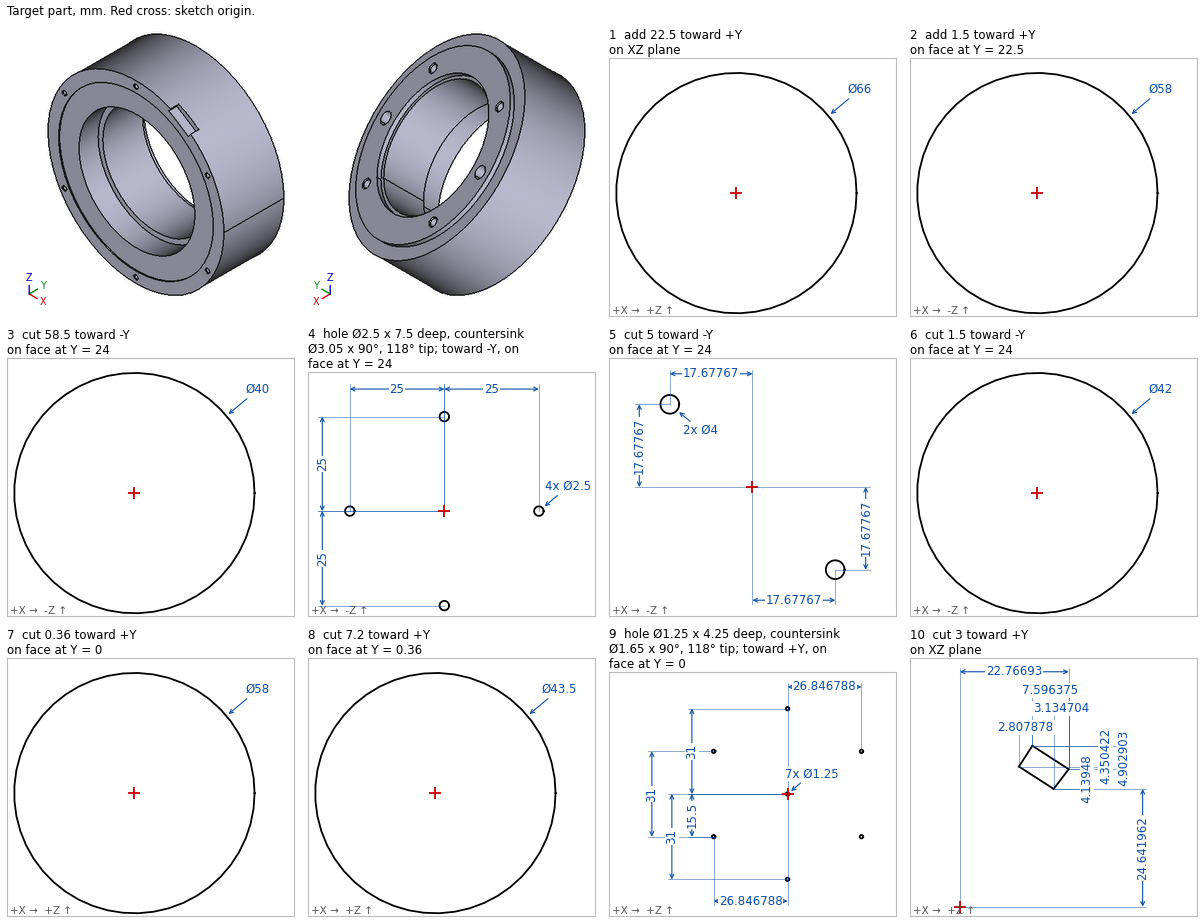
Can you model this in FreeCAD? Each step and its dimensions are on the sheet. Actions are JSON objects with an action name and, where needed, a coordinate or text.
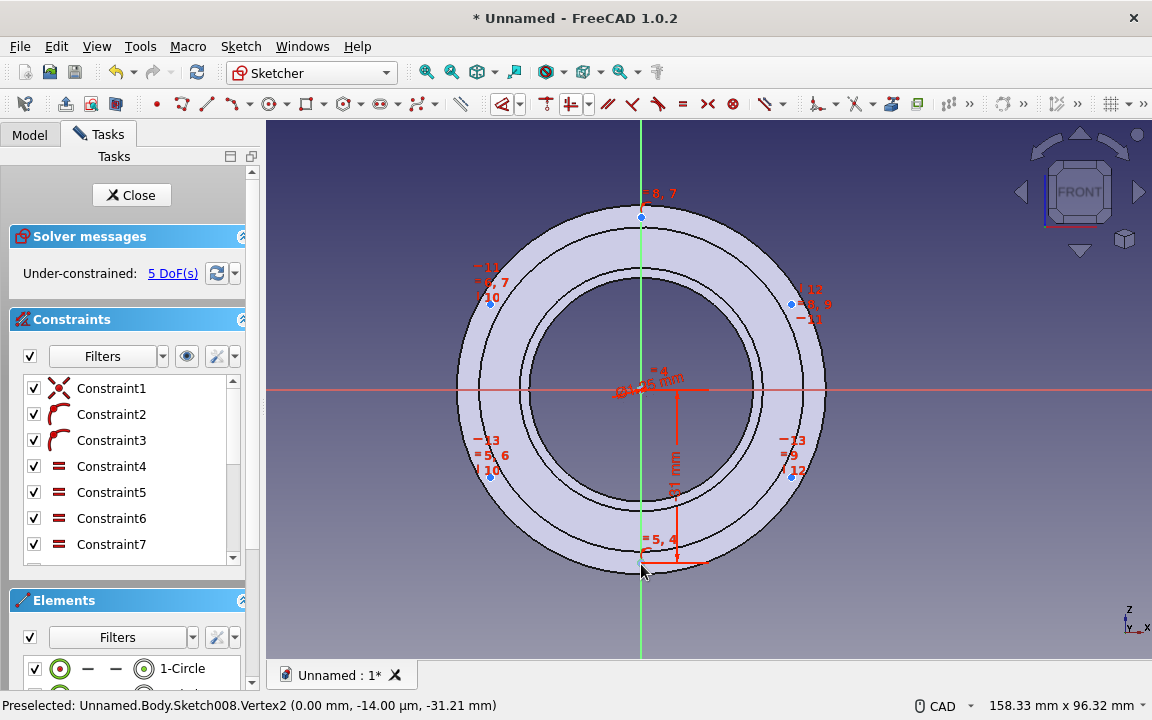
{"action": "left_click", "coordinate": [641, 217]}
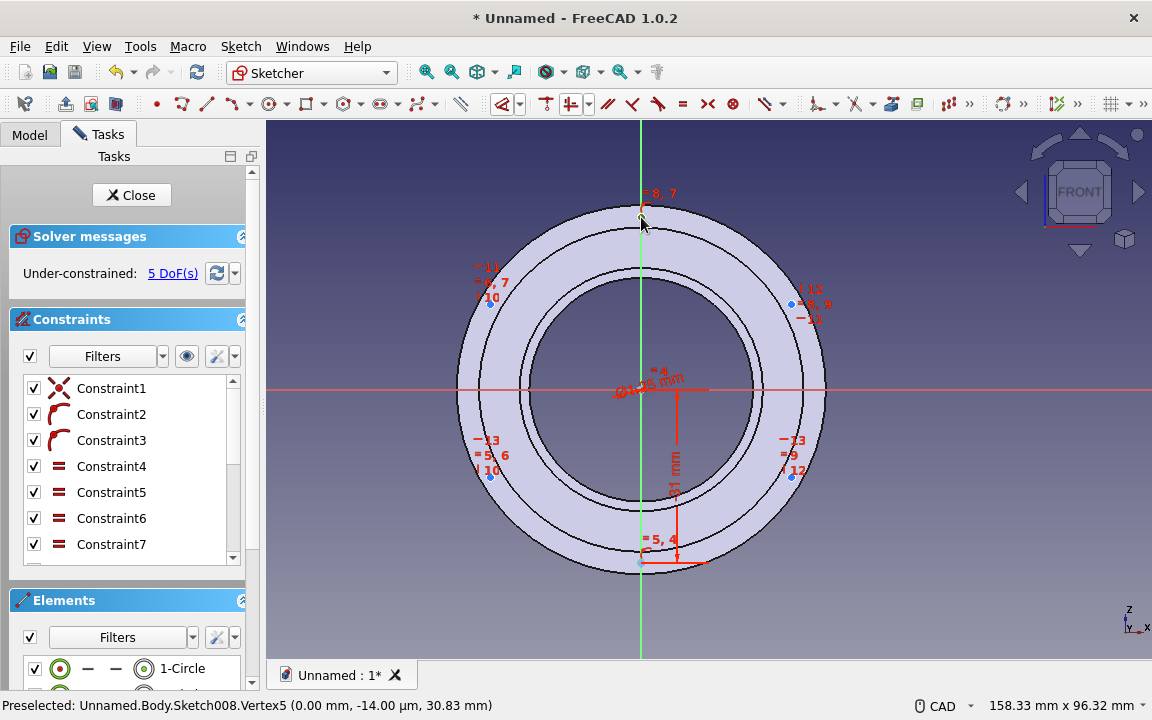
{"action": "key", "text": "i"}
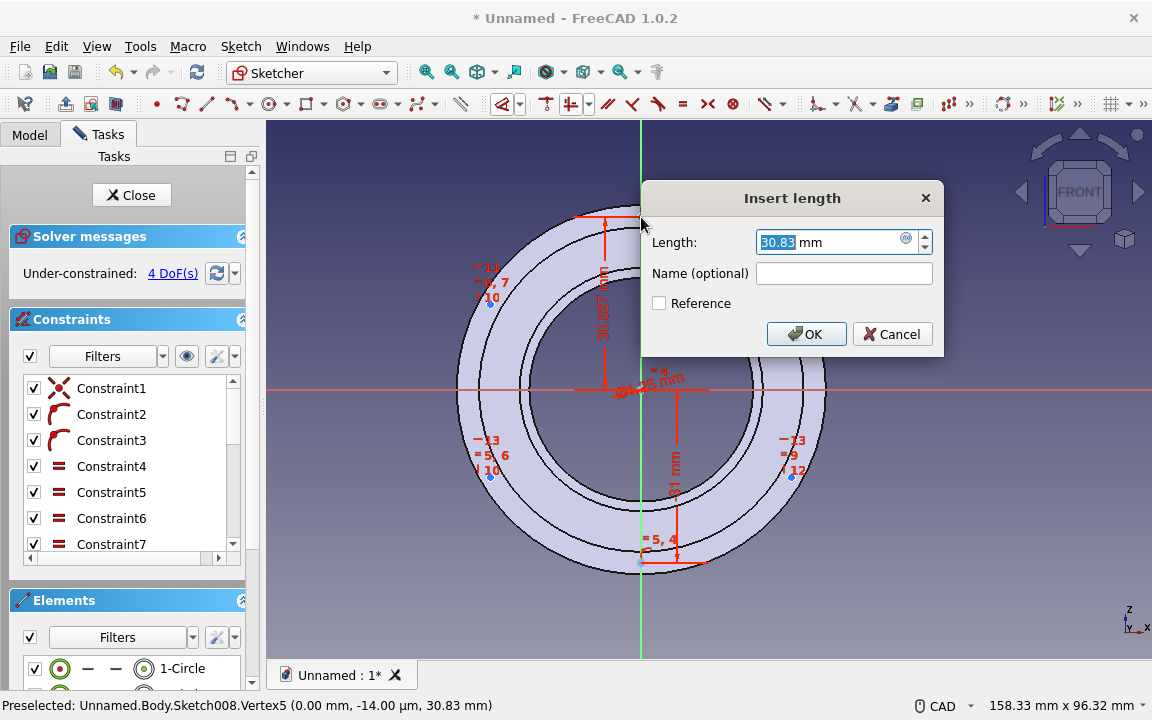
{"action": "type", "text": "31"}
{"action": "key", "text": "Return"}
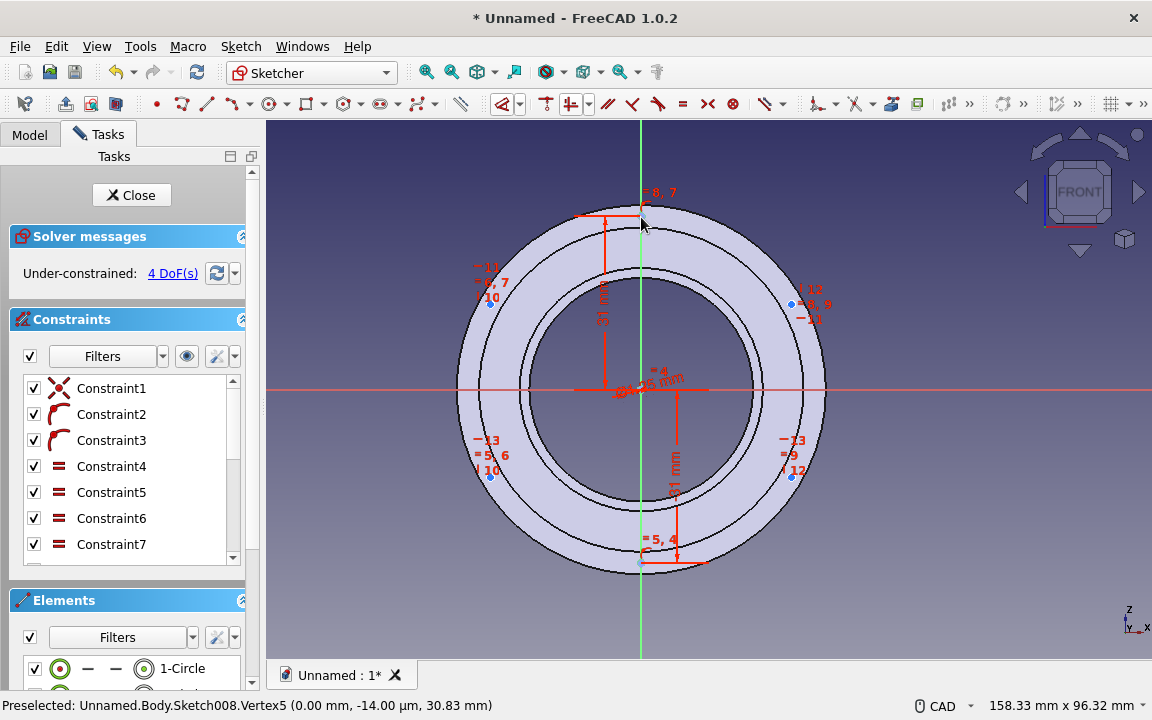
{"action": "left_click", "coordinate": [491, 477]}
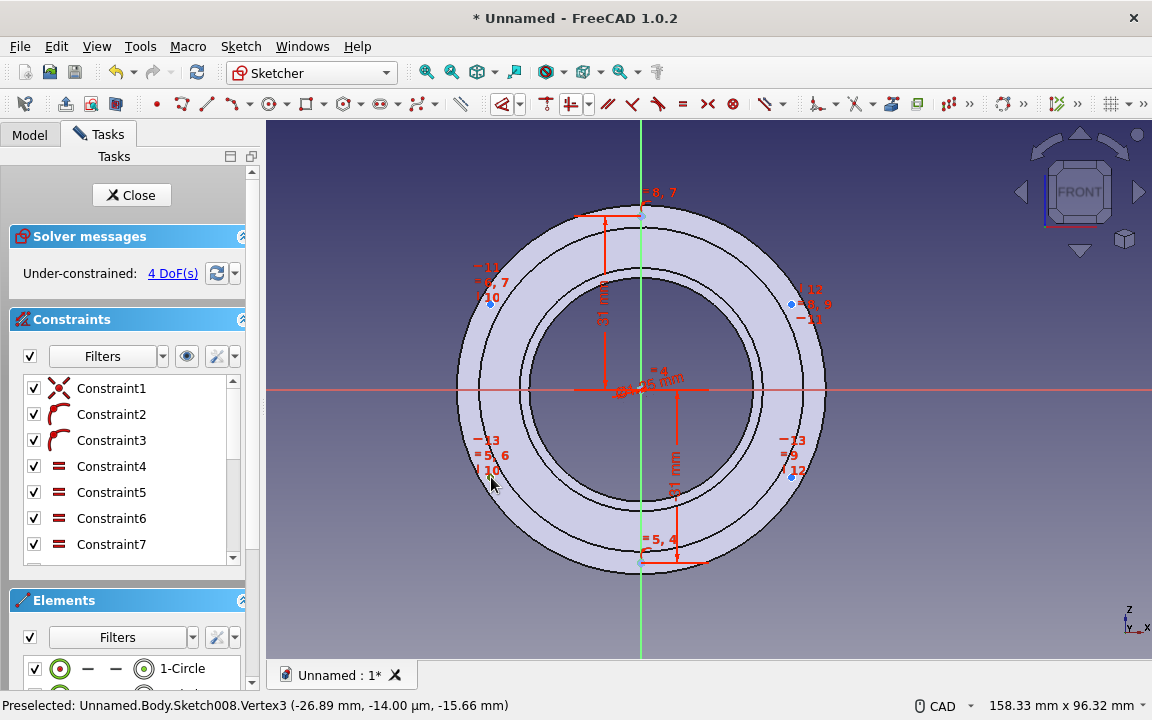
{"action": "left_click", "coordinate": [491, 304]}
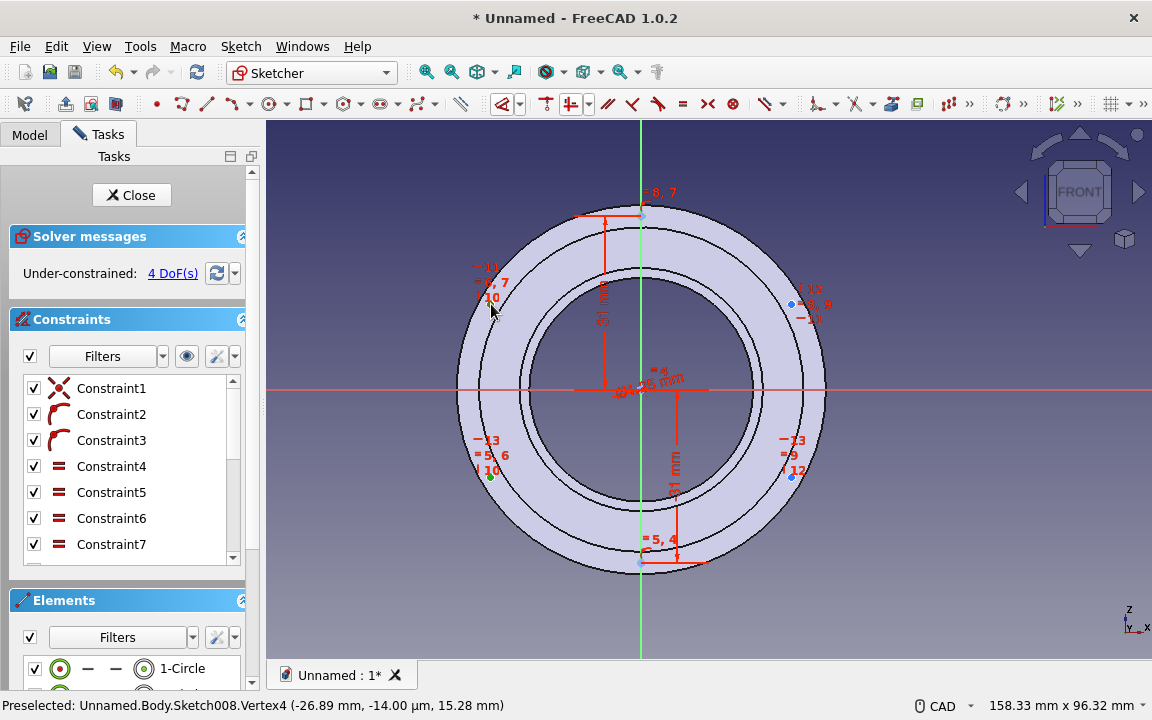
{"action": "key", "text": "i"}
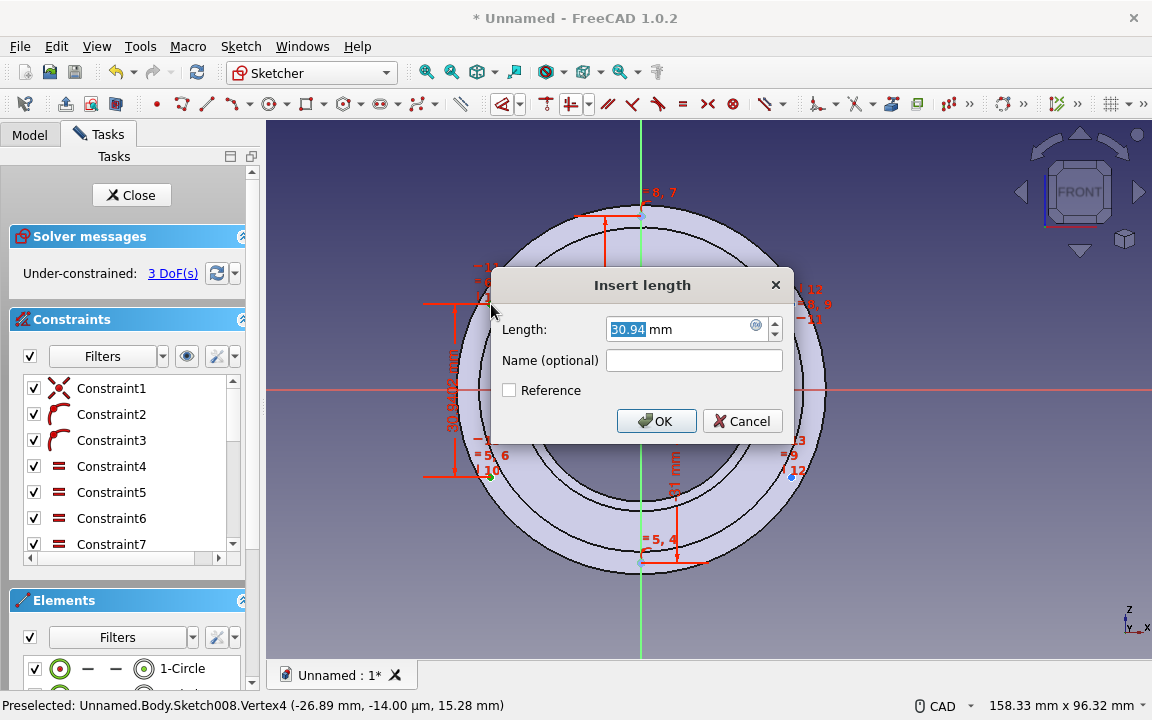
{"action": "type", "text": "31"}
{"action": "key", "text": "Return"}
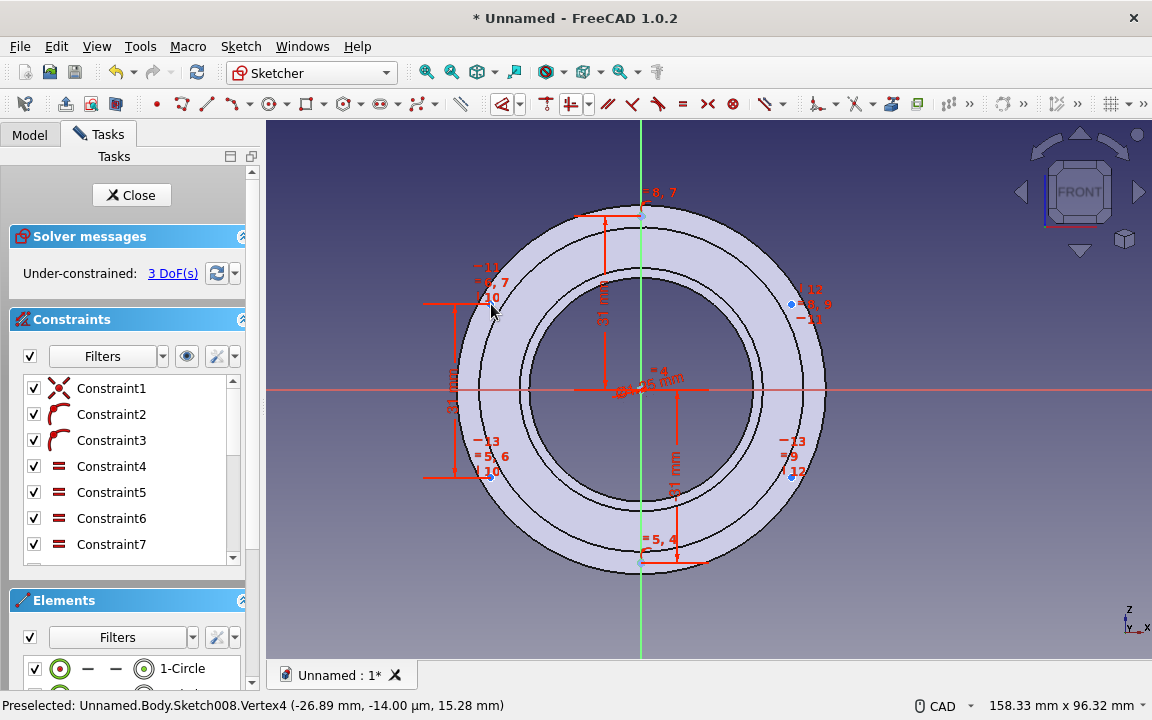
{"action": "left_click", "coordinate": [491, 478]}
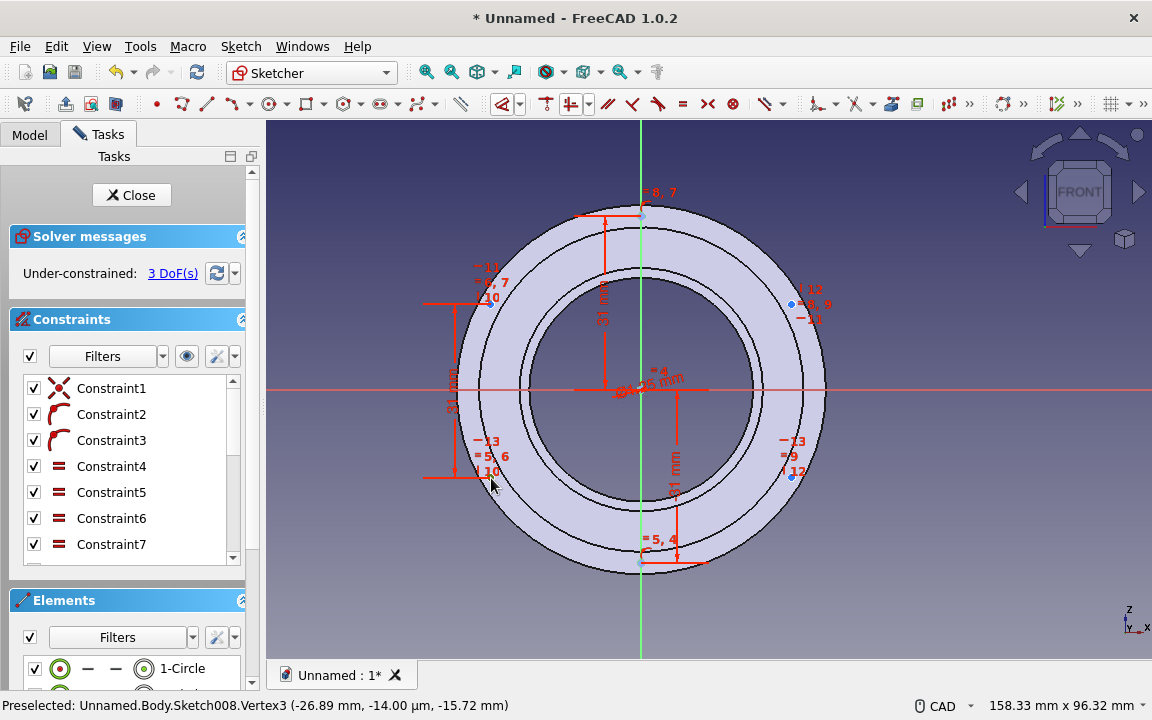
{"action": "left_click", "coordinate": [520, 104]}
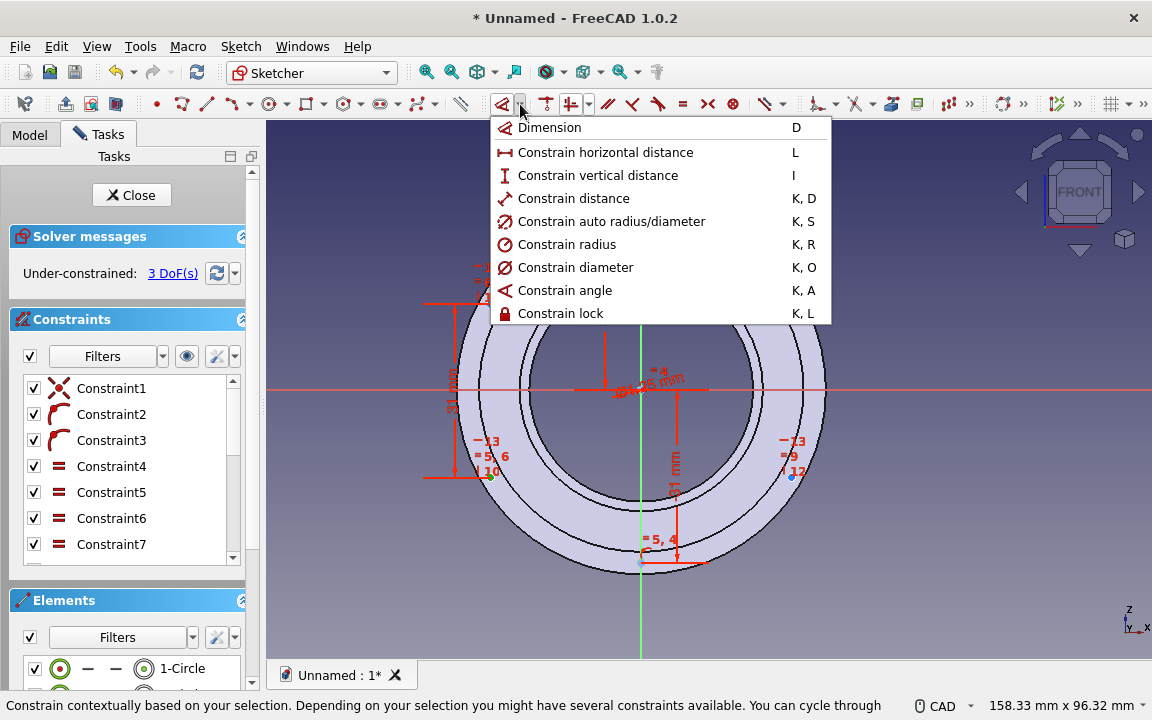
{"action": "left_click", "coordinate": [661, 176]}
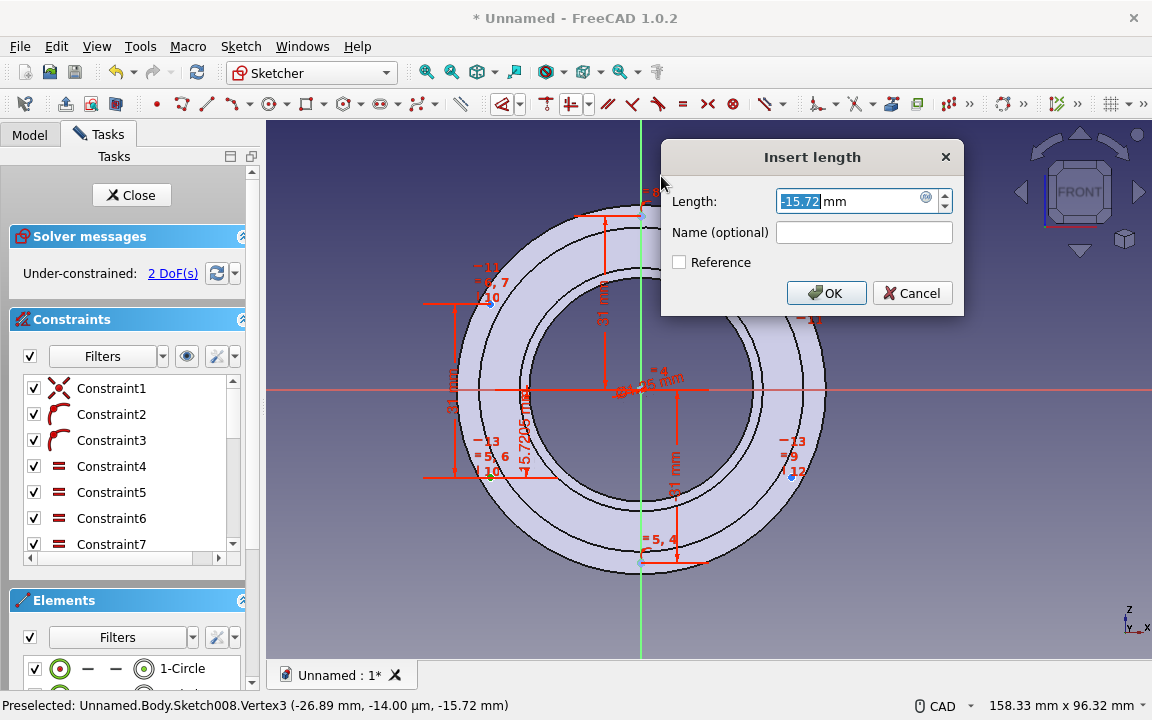
{"action": "type", "text": "-15.5"}
{"action": "key", "text": "Return"}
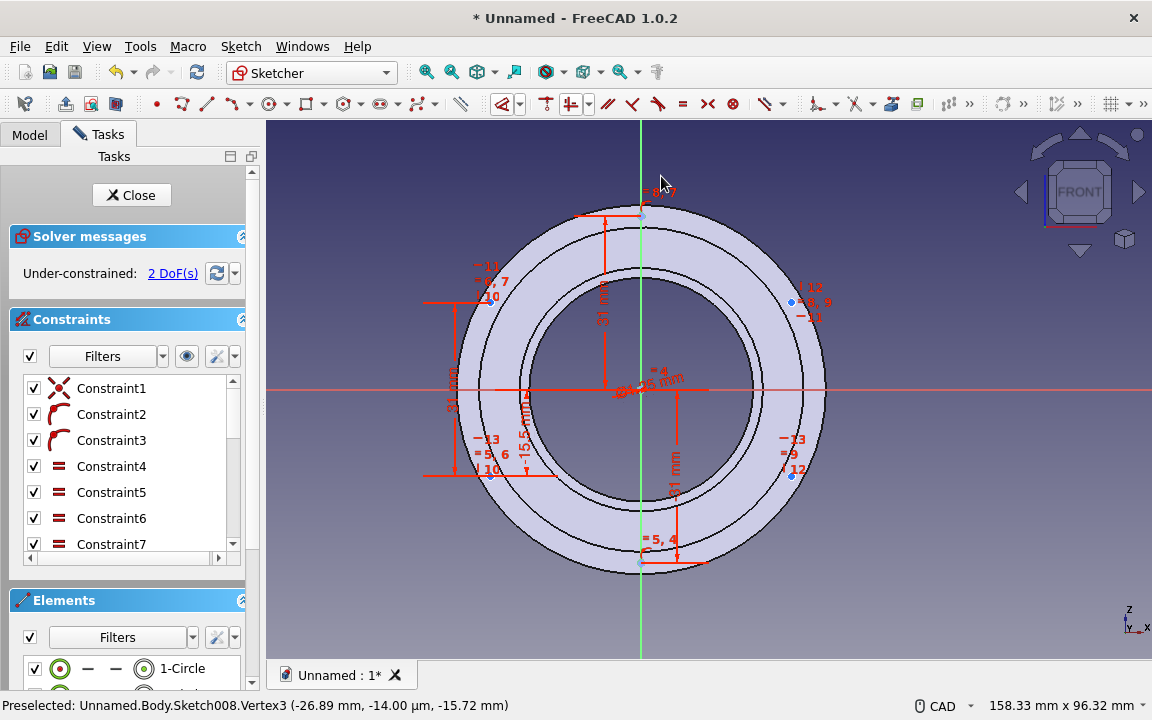
{"action": "left_click", "coordinate": [491, 476]}